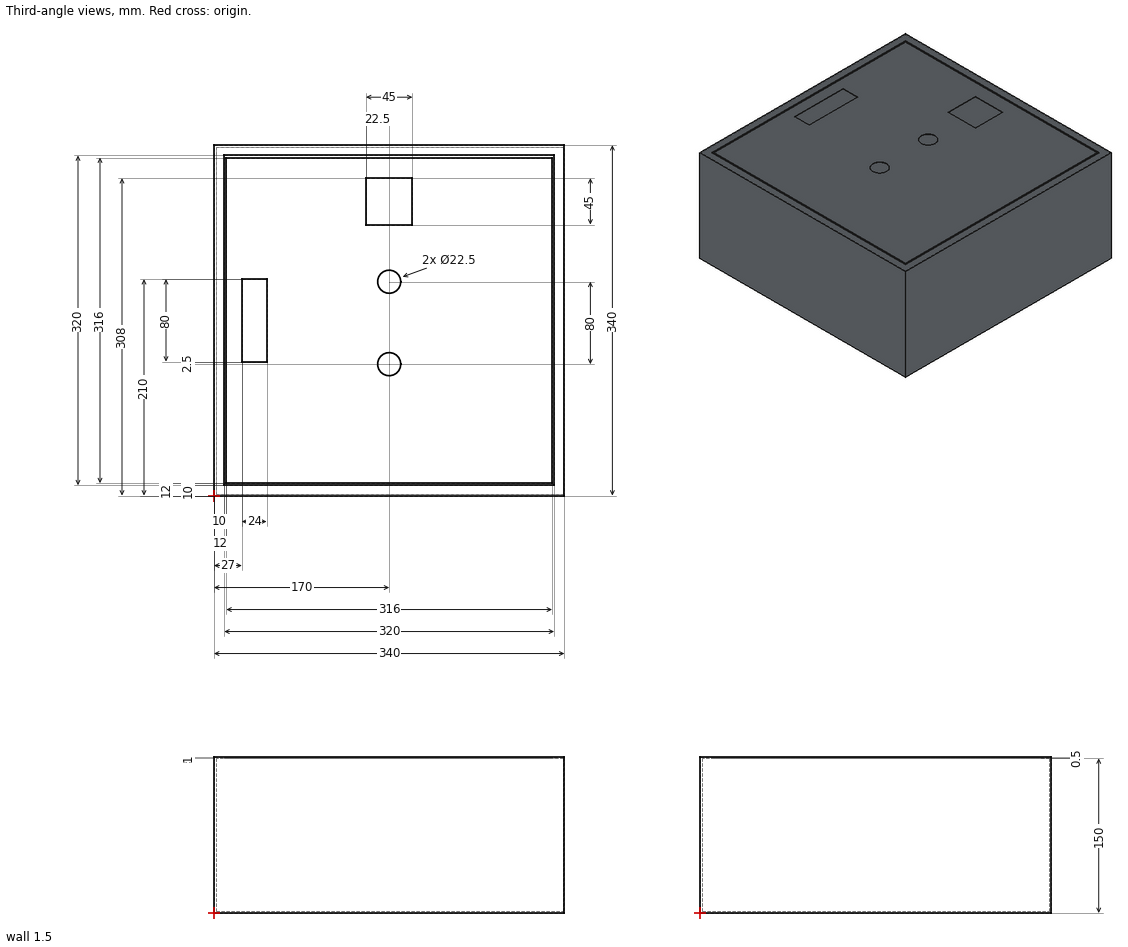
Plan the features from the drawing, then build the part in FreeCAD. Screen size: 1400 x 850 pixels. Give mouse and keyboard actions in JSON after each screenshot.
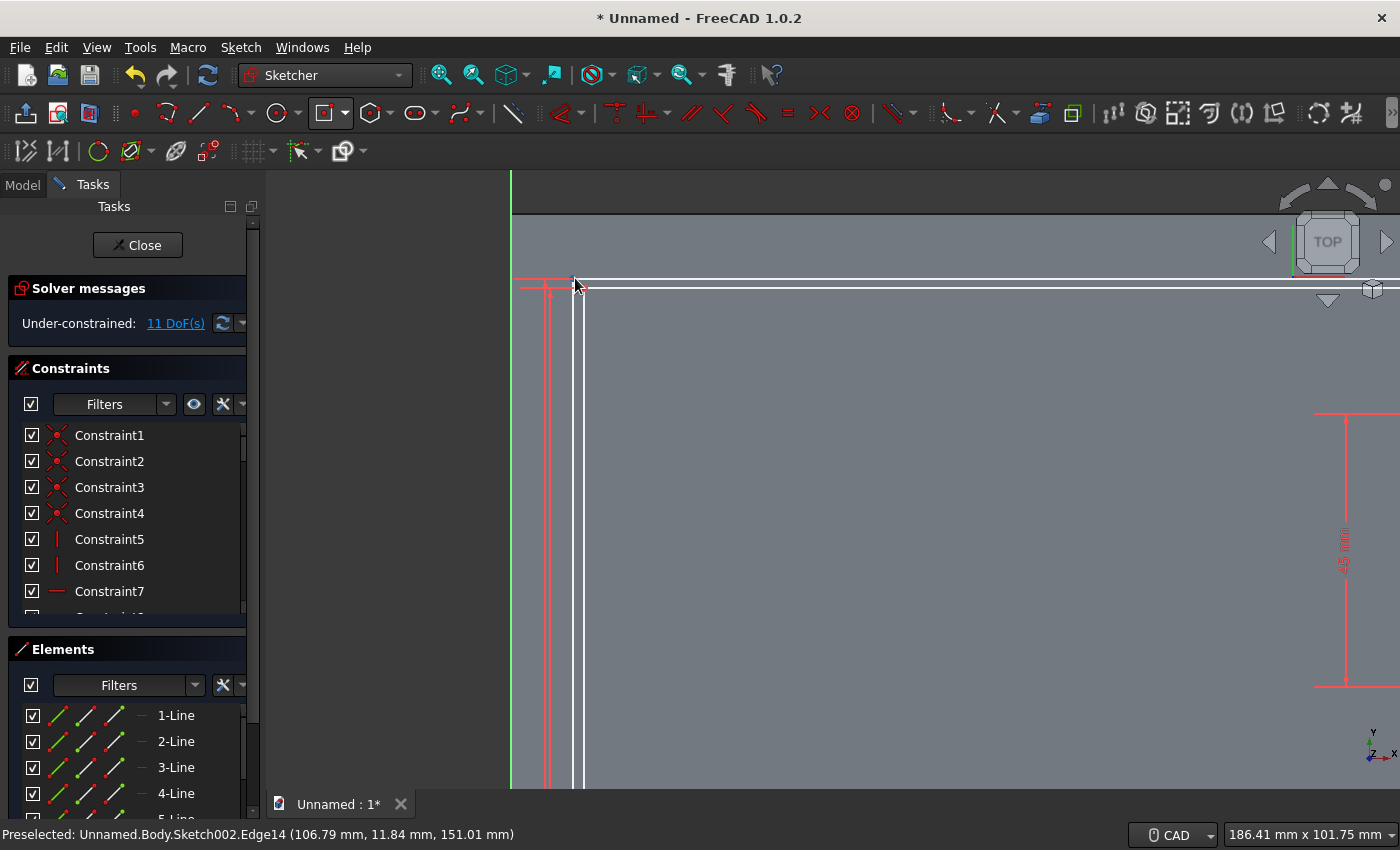
{"action": "left_click", "coordinate": [573, 279]}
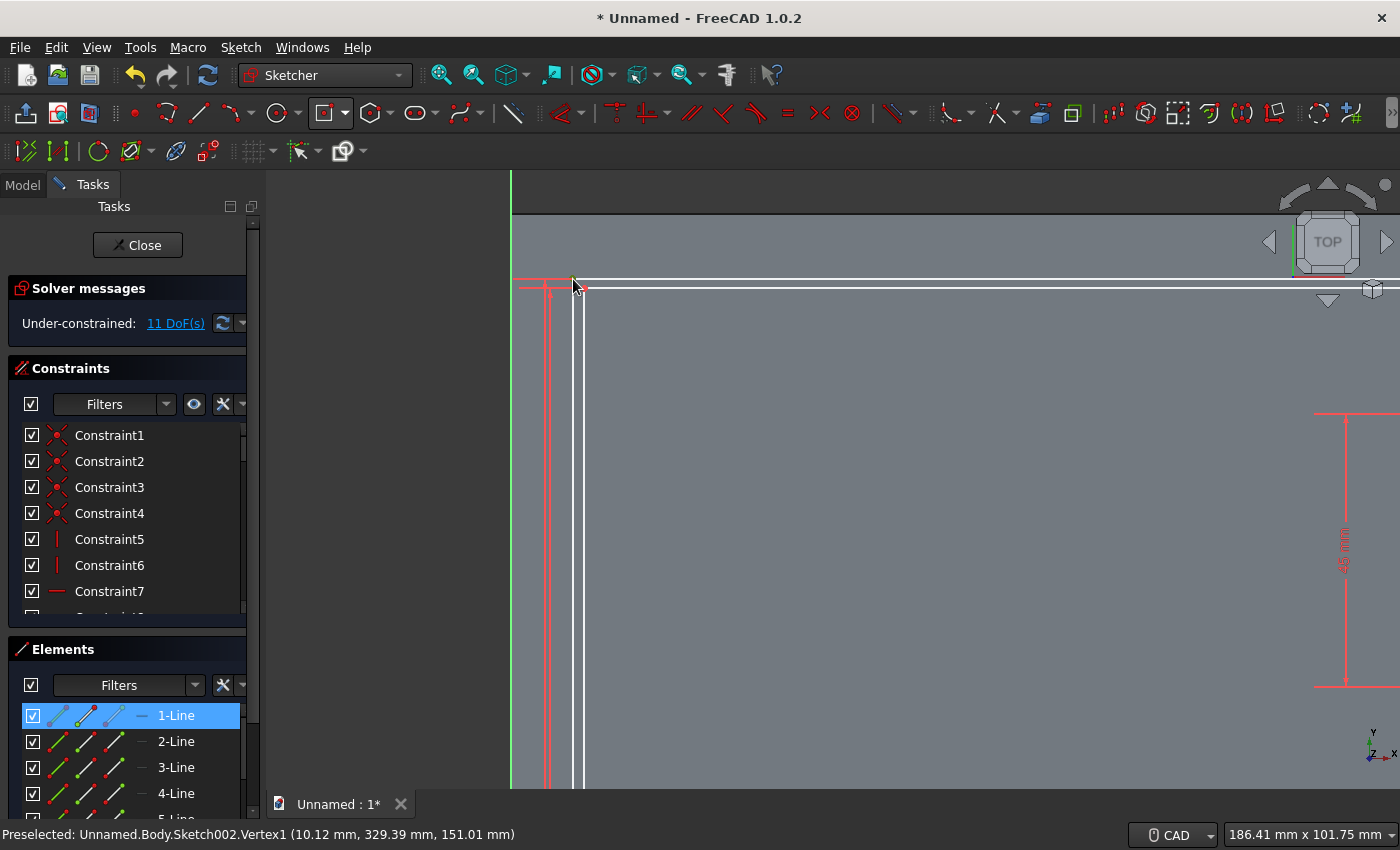
{"action": "key", "text": "l"}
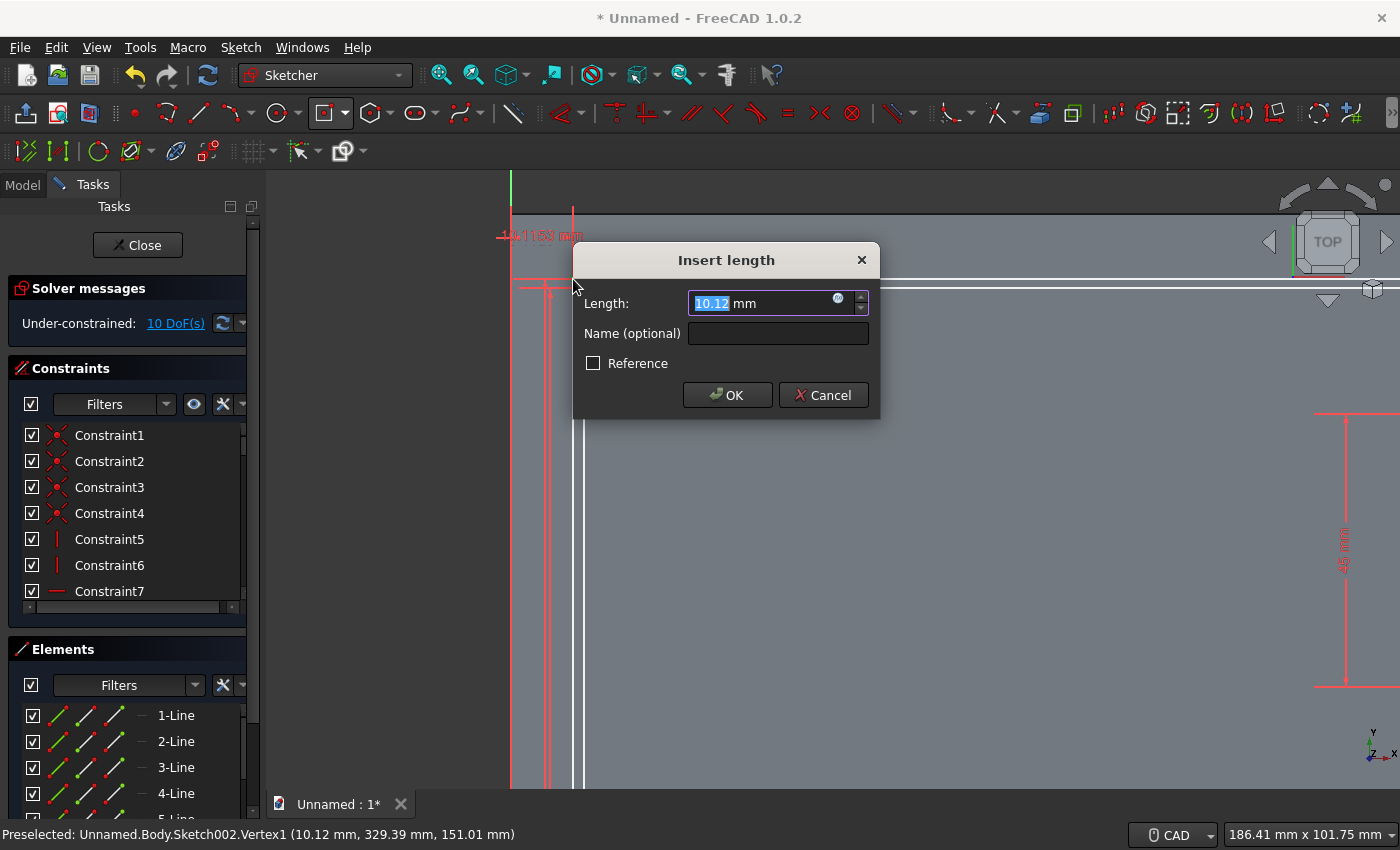
{"action": "type", "text": "10"}
{"action": "key", "text": "Return"}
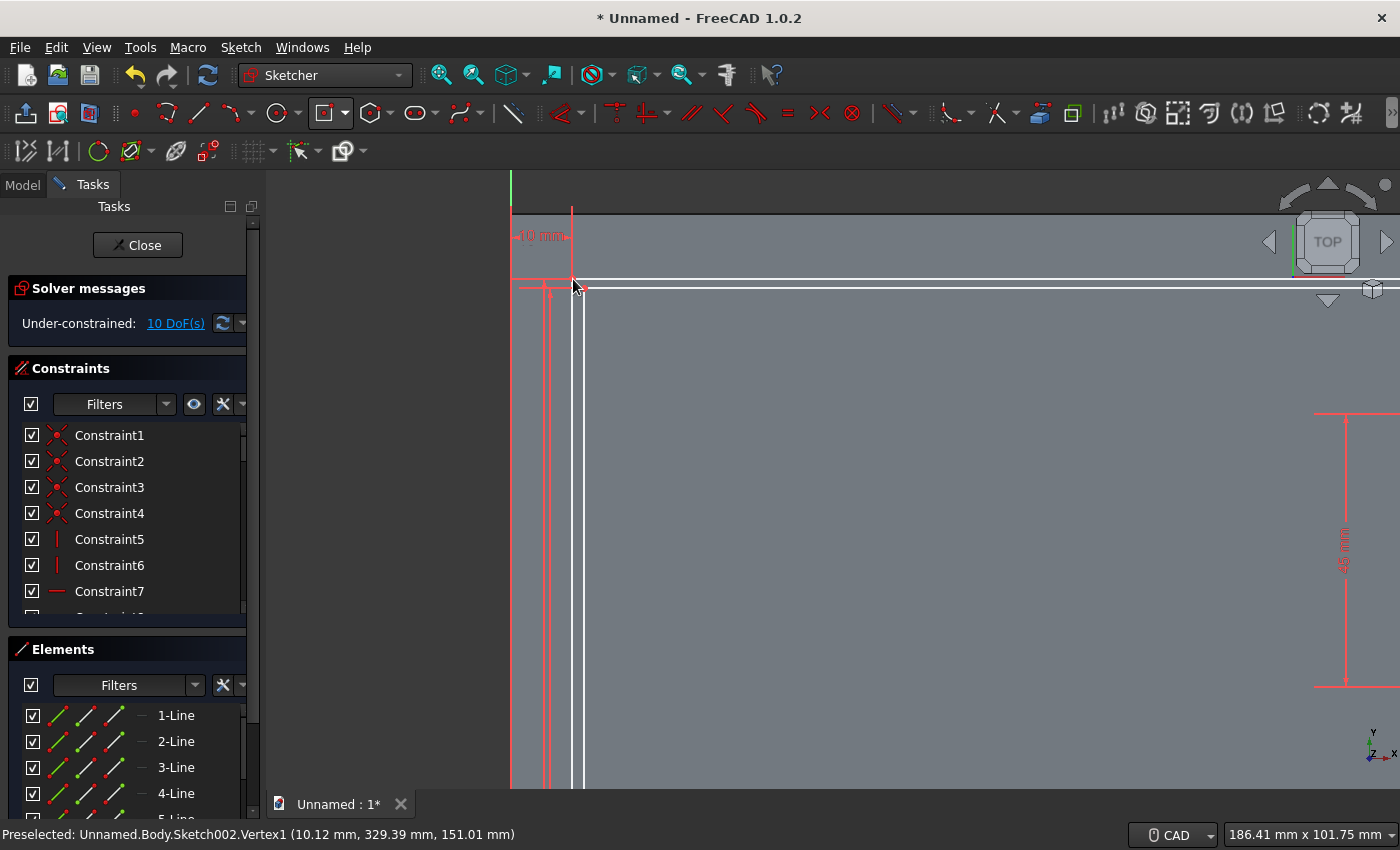
{"action": "scroll", "coordinate": [575, 277], "scroll_direction": "down", "scroll_amount": 8}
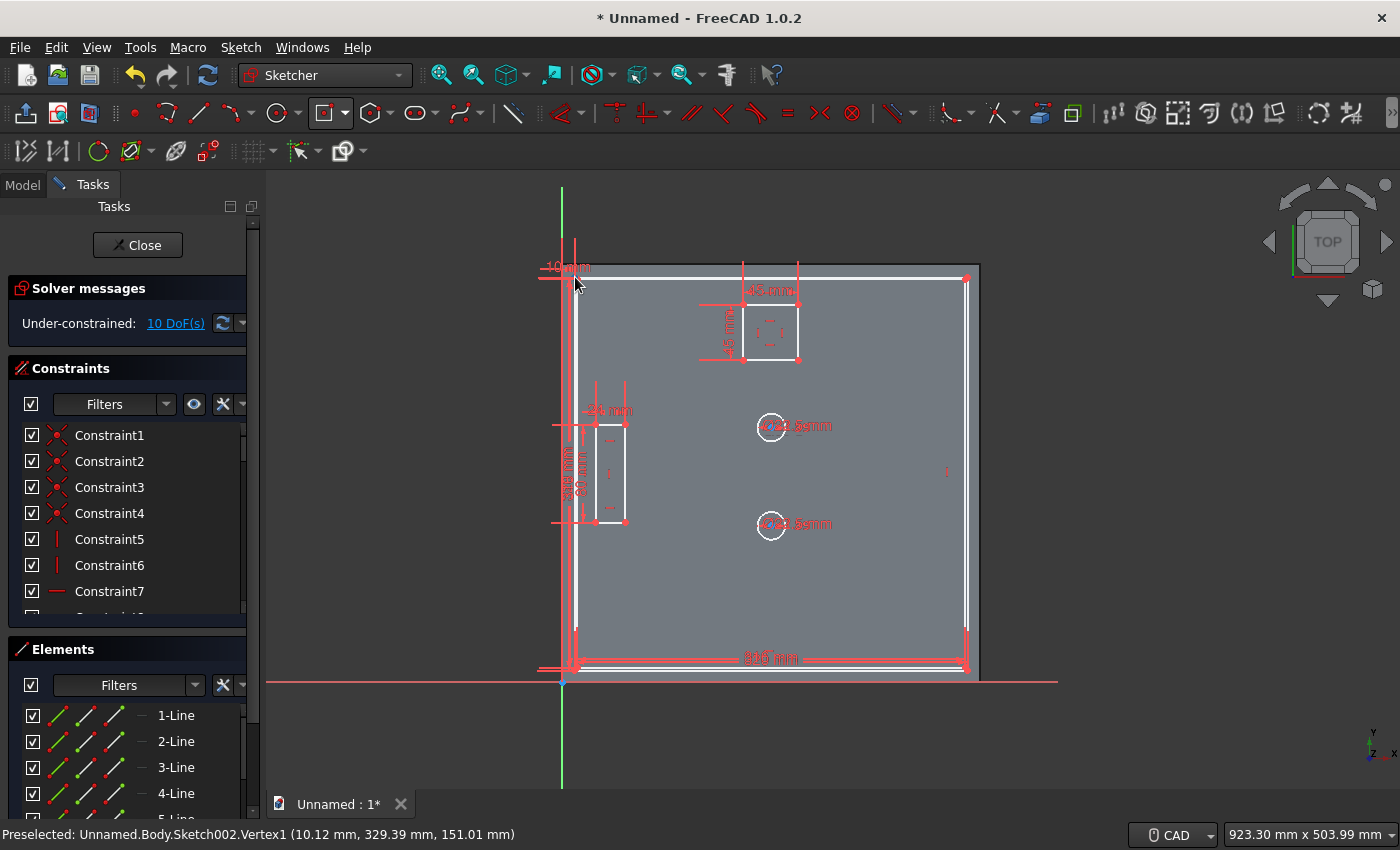
{"action": "scroll", "coordinate": [575, 671], "scroll_direction": "up", "scroll_amount": 6}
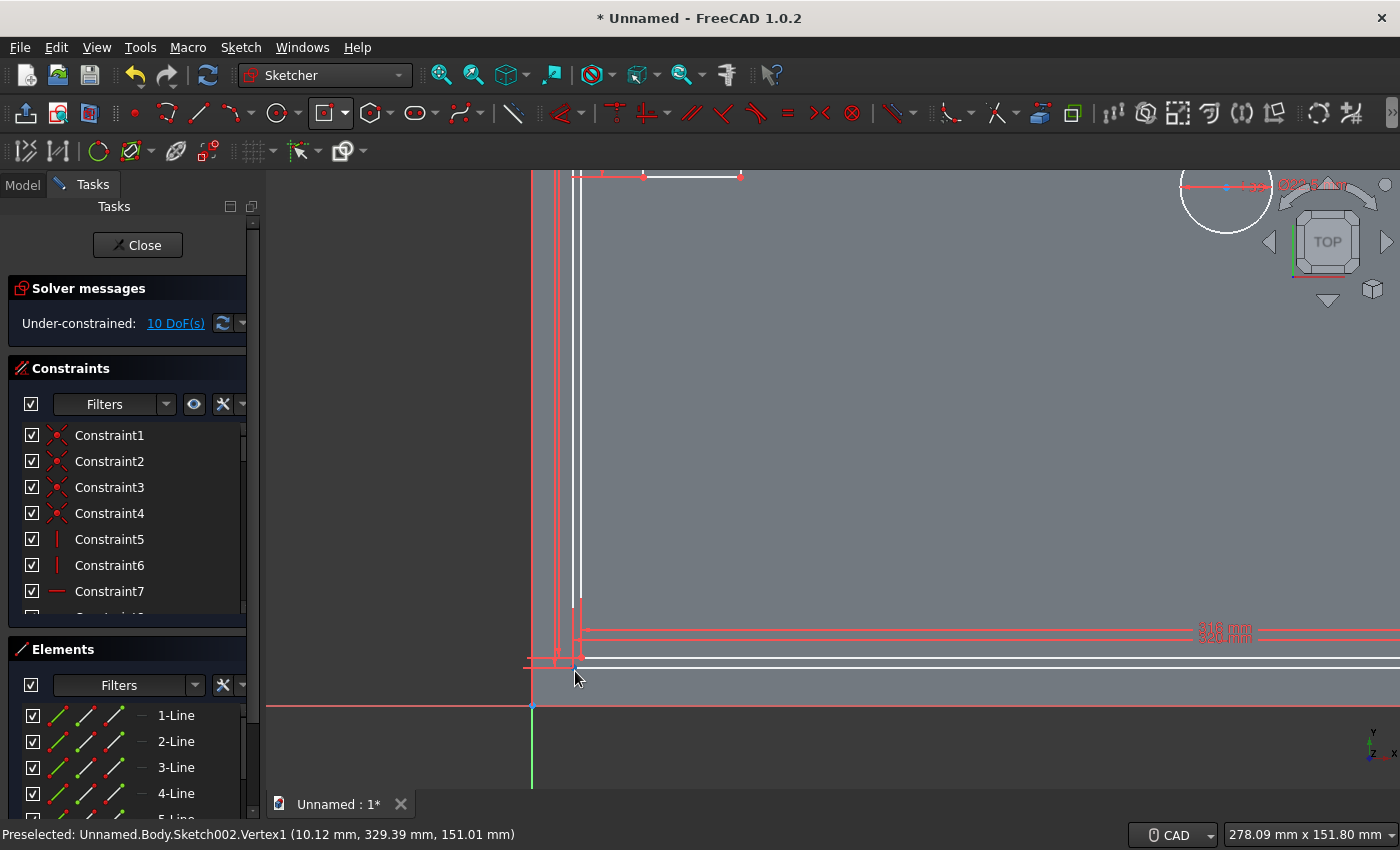
{"action": "left_click", "coordinate": [573, 668]}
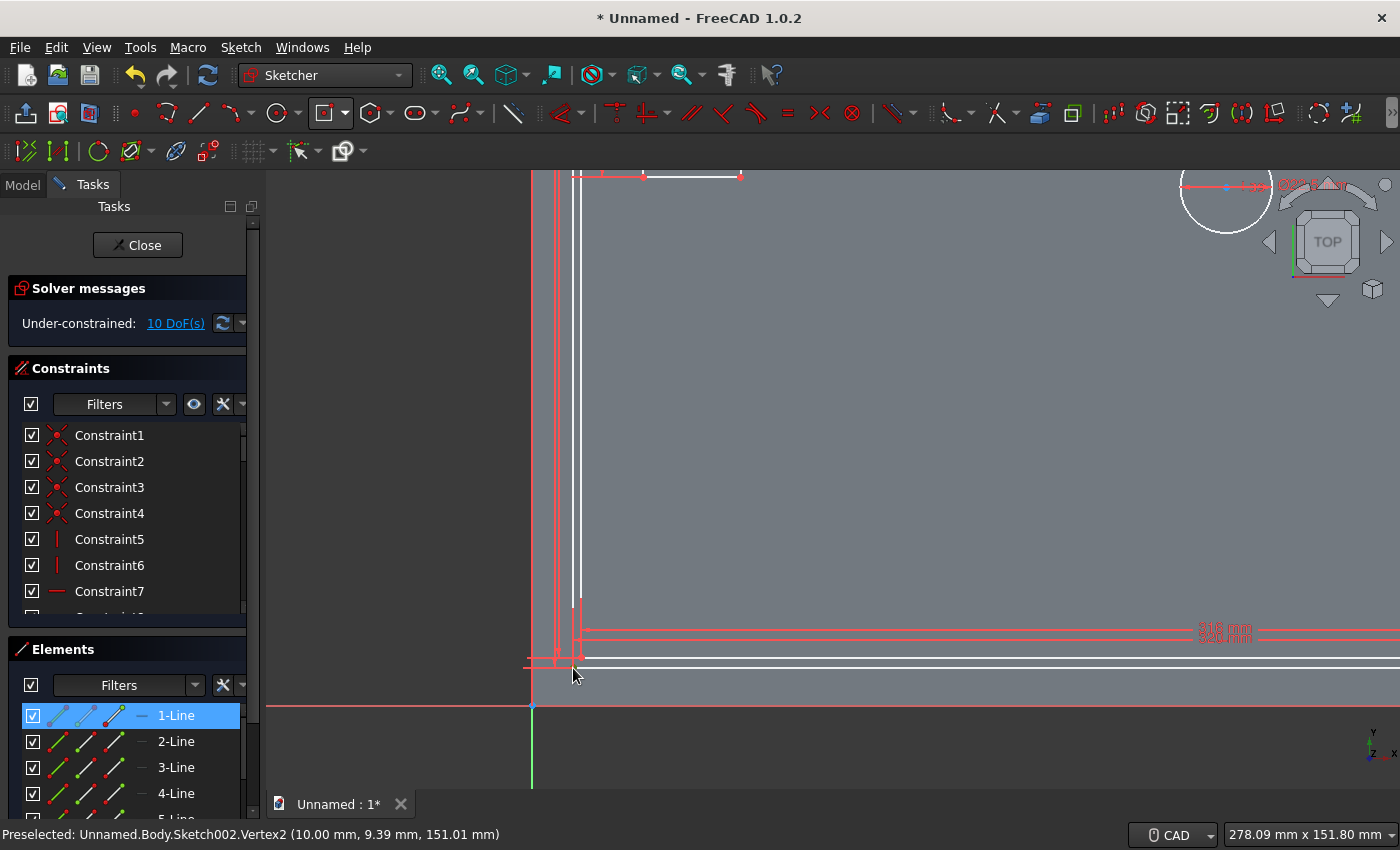
{"action": "key", "text": "i"}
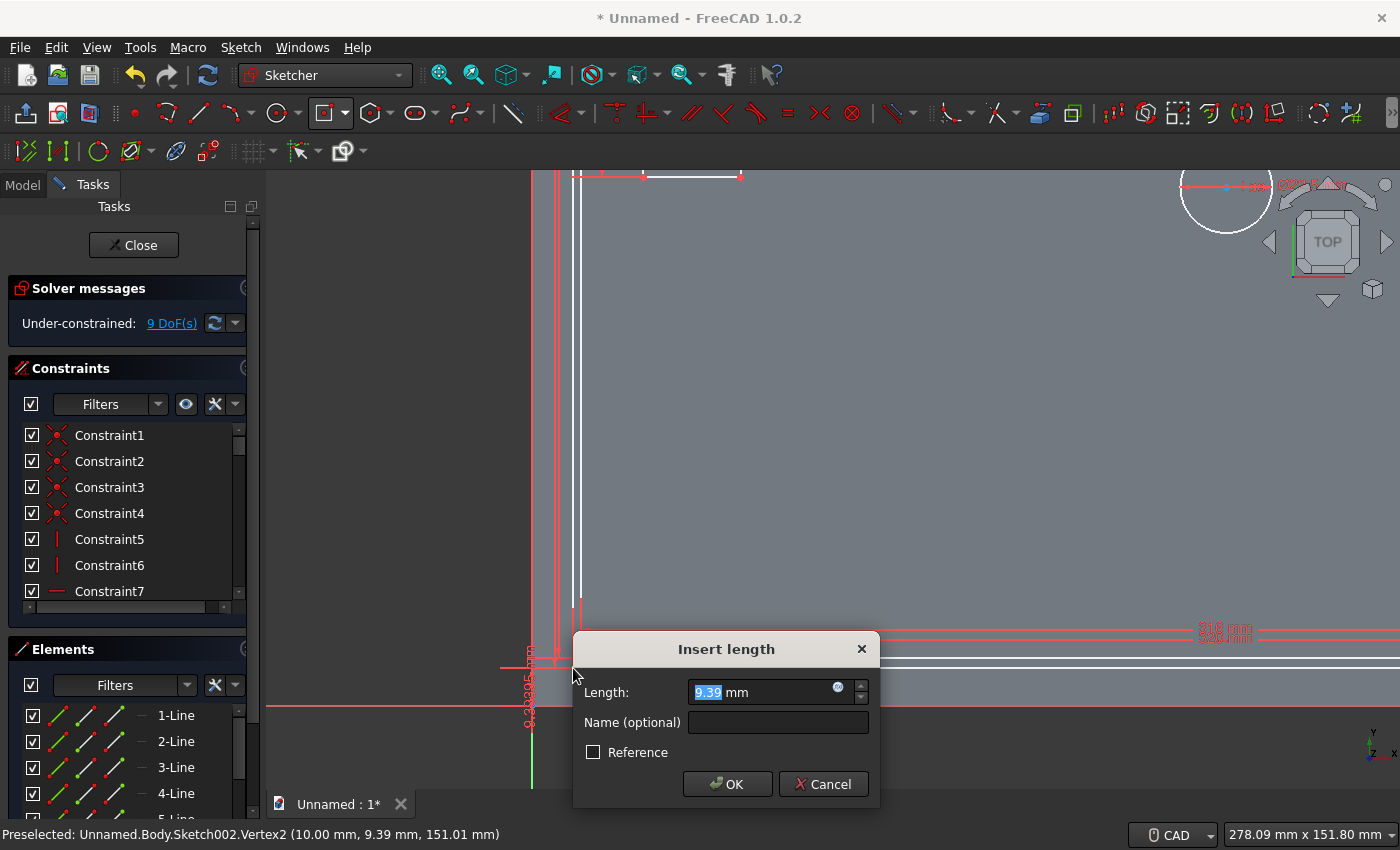
{"action": "type", "text": "10"}
{"action": "key", "text": "Return"}